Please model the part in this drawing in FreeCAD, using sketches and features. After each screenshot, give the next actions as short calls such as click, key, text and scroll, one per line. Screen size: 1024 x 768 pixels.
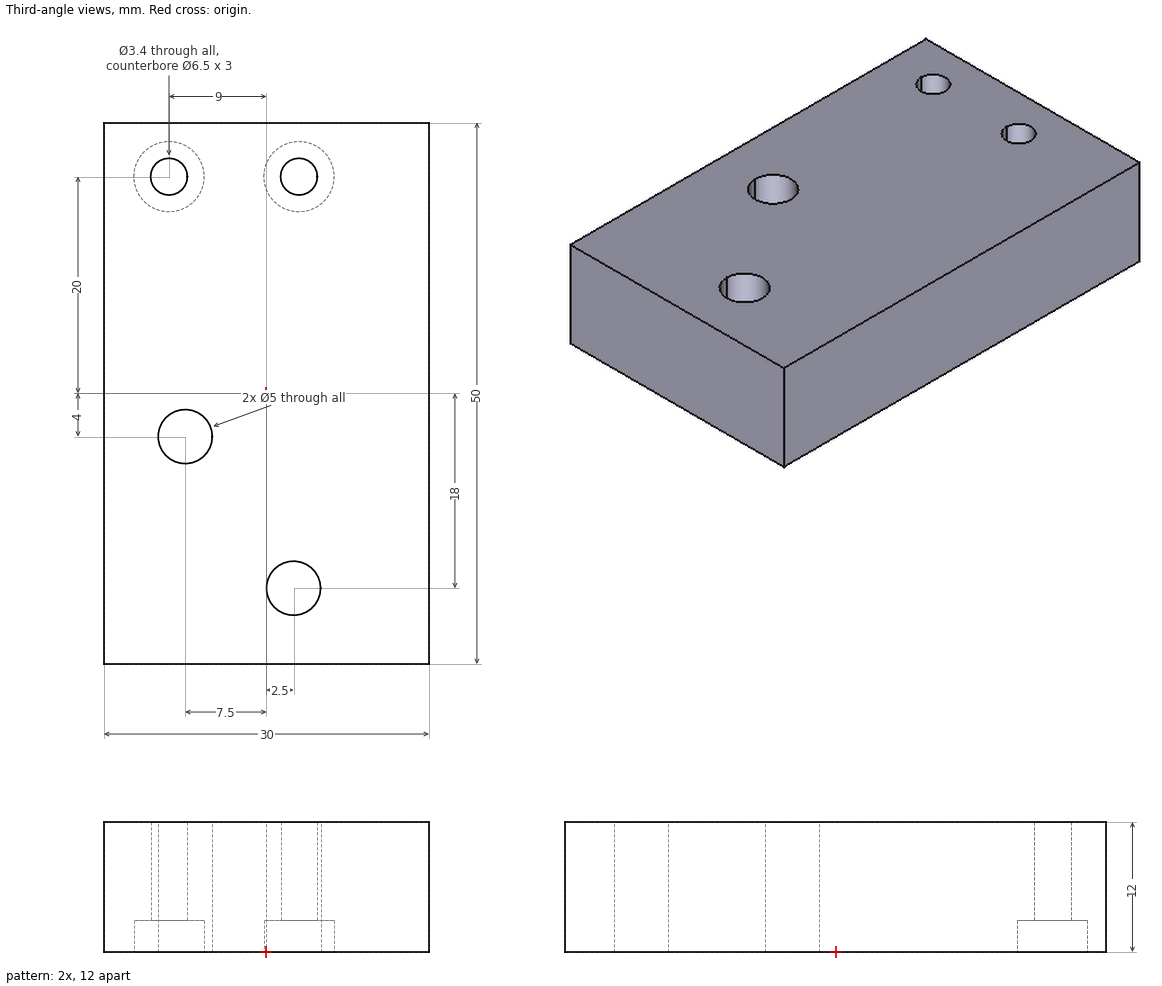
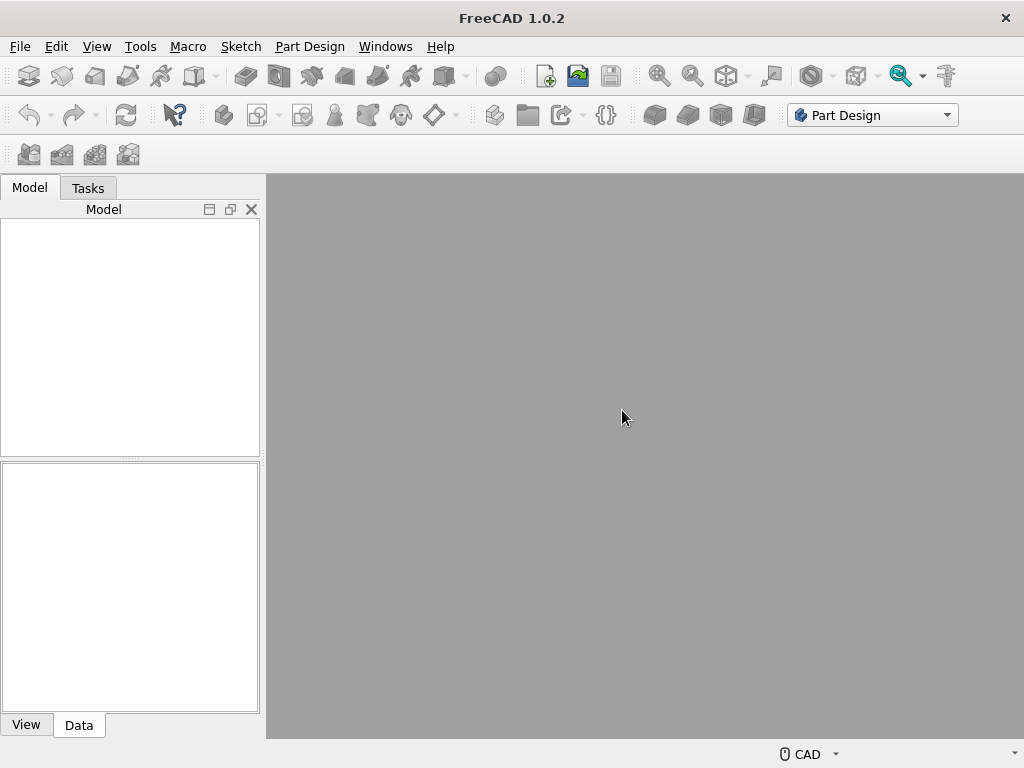
key(ctrl+n)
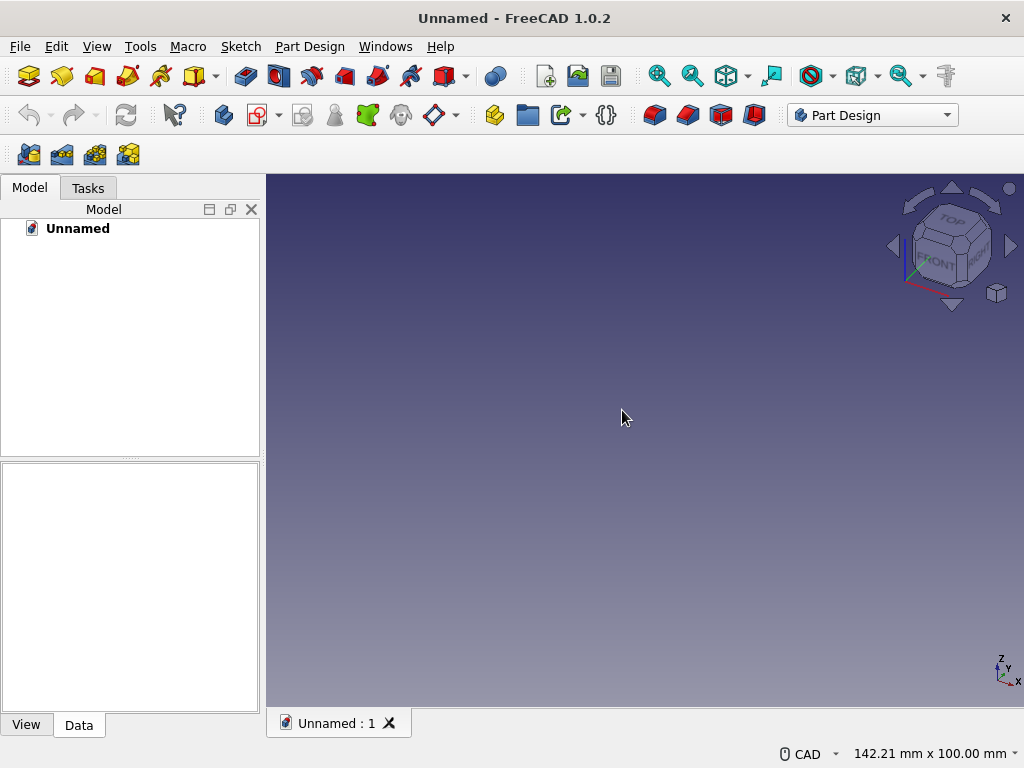
click(256, 116)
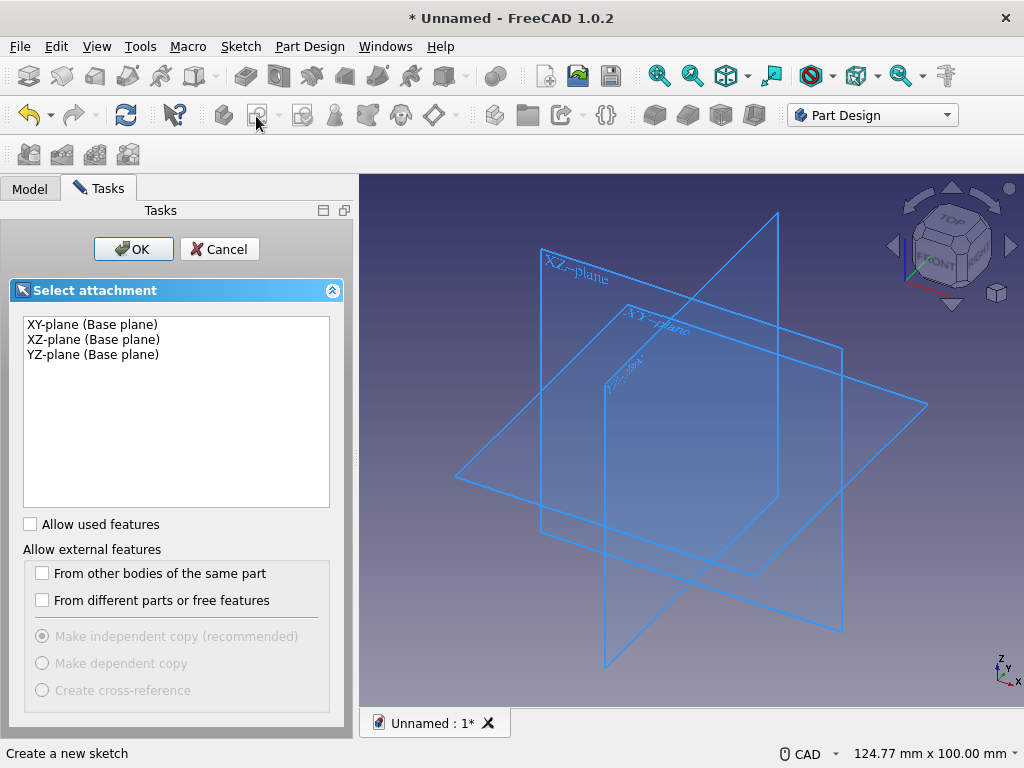
click(84, 324)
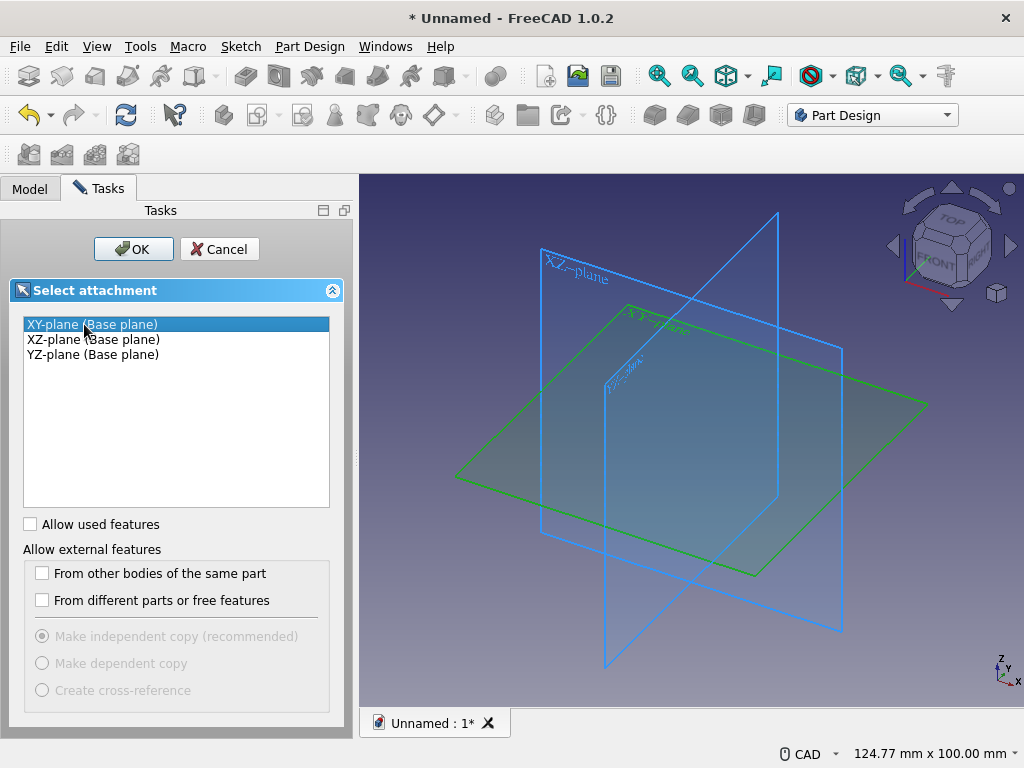
click(134, 249)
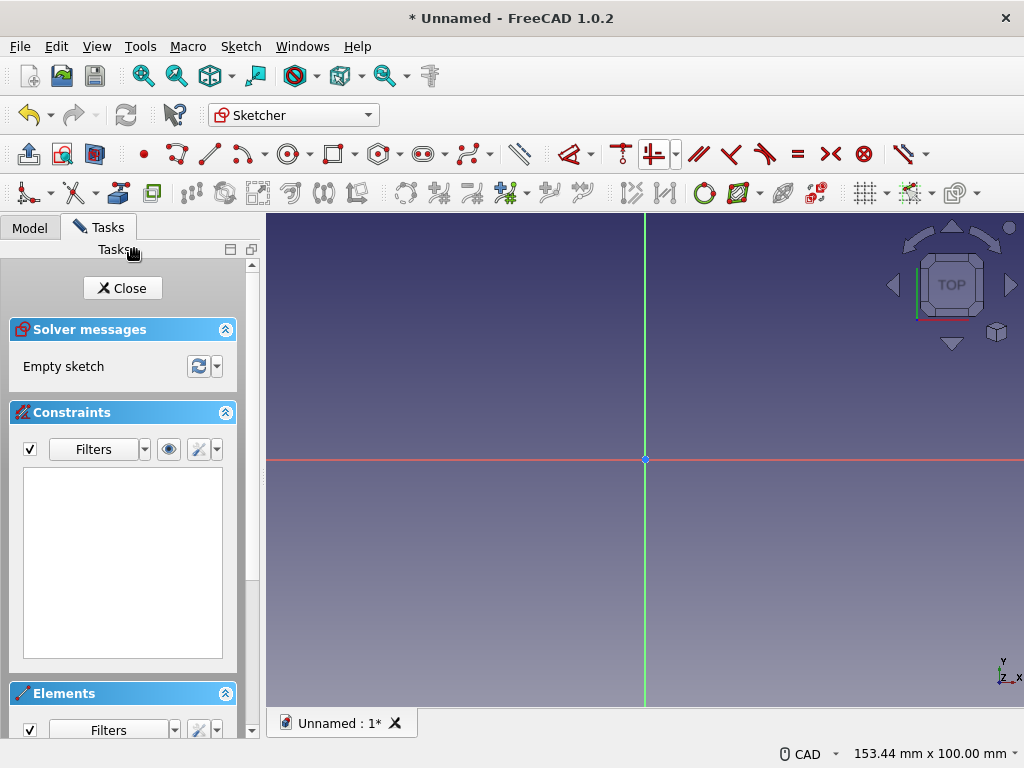
key(g)
key(v)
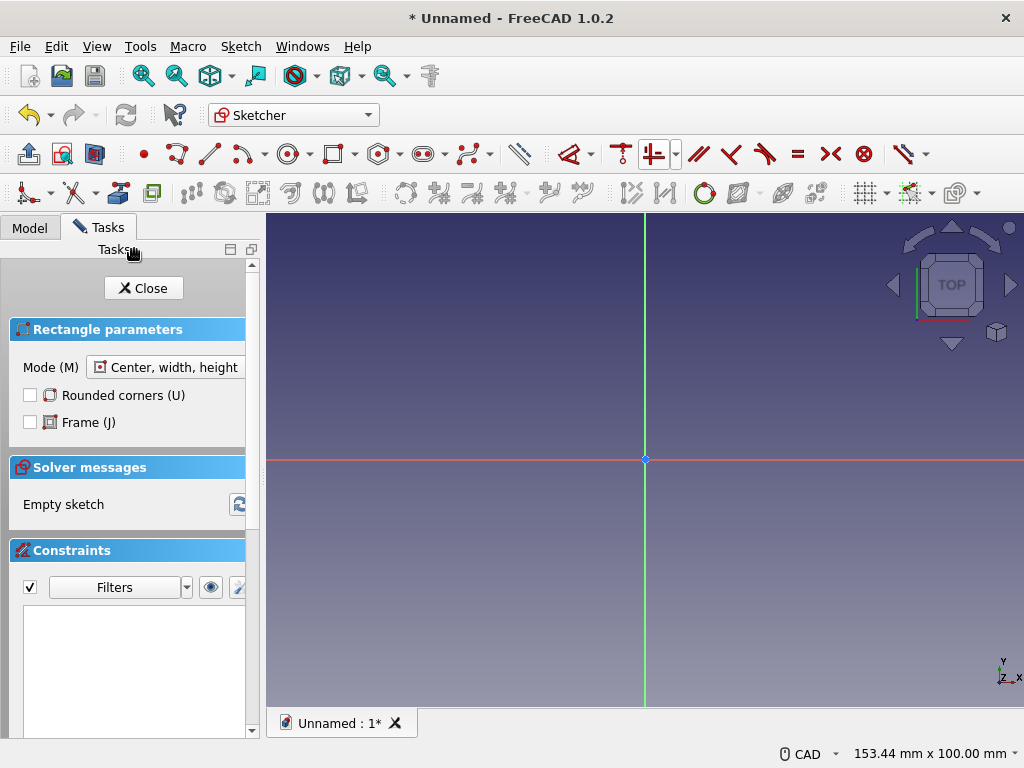
click(645, 460)
move(719, 336)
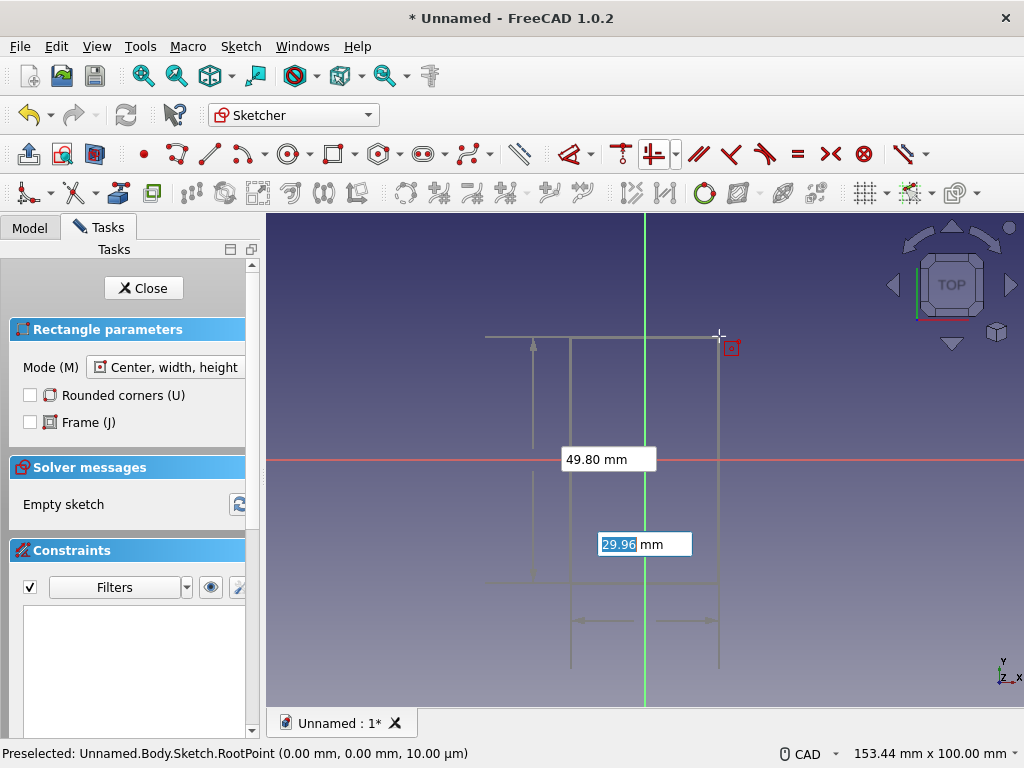
text(30)
key(Tab)
text(50)
key(Return)
key(Escape)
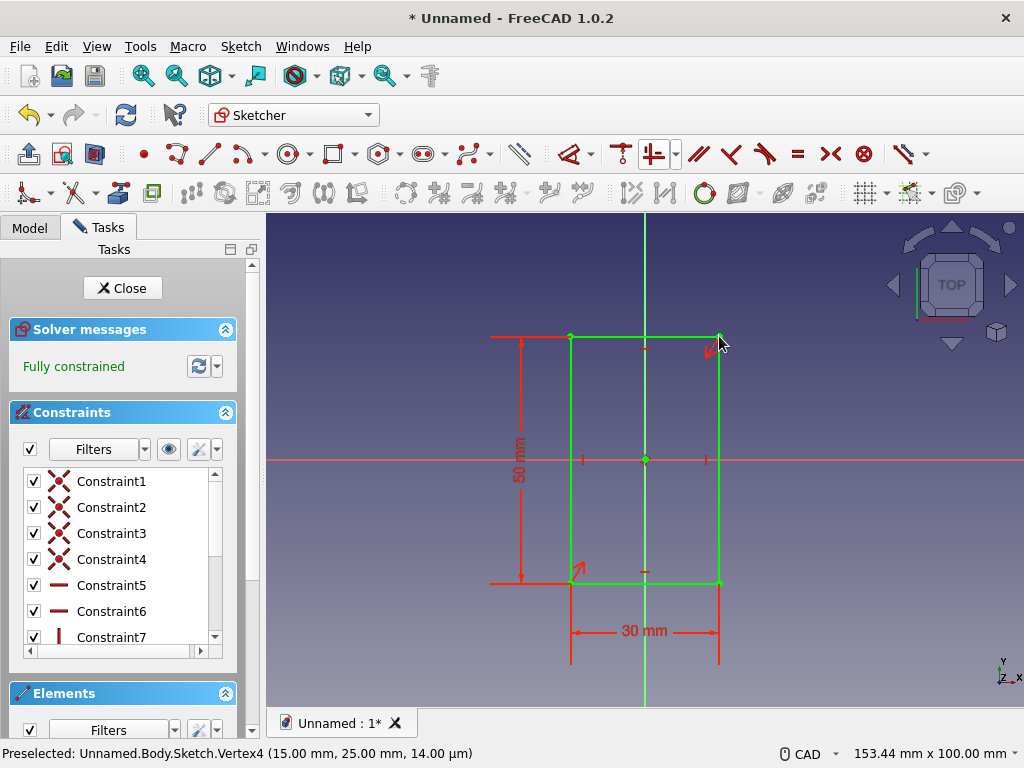
click(123, 288)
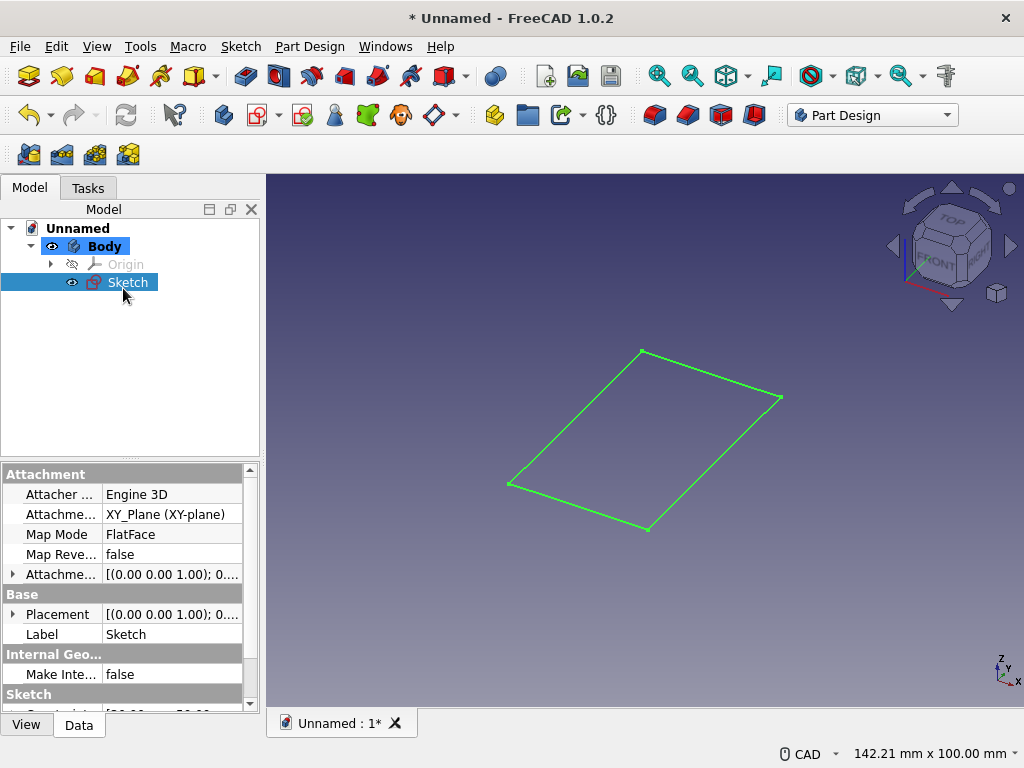
click(29, 76)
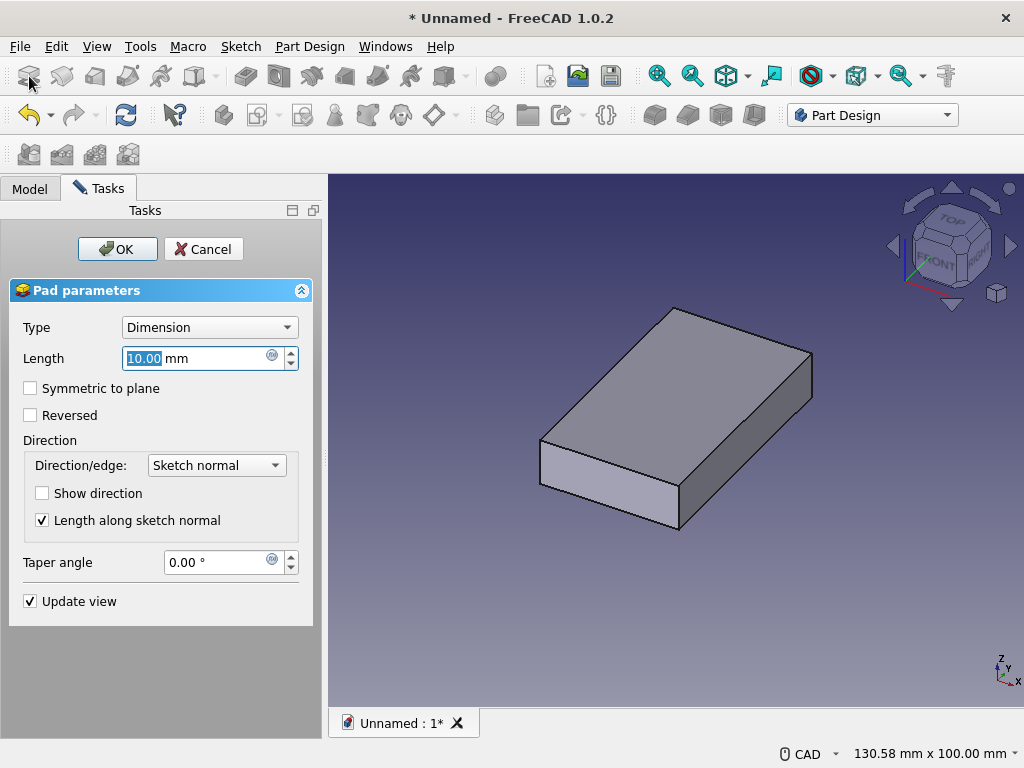
text(12)
key(Tab)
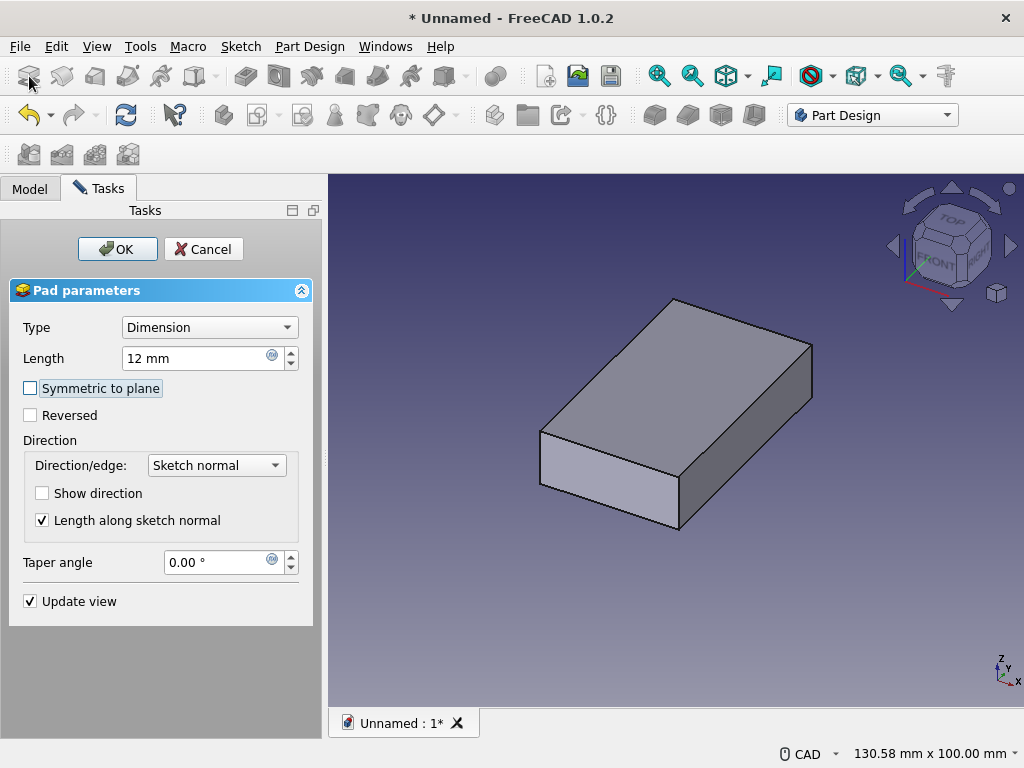
click(118, 249)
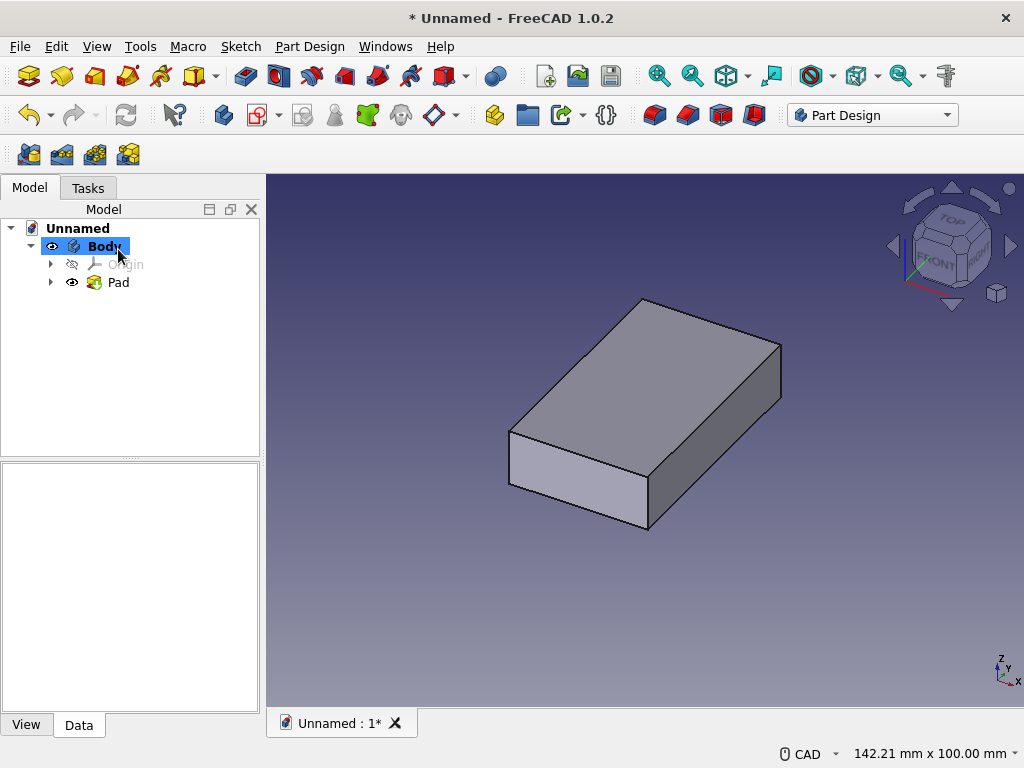
click(660, 76)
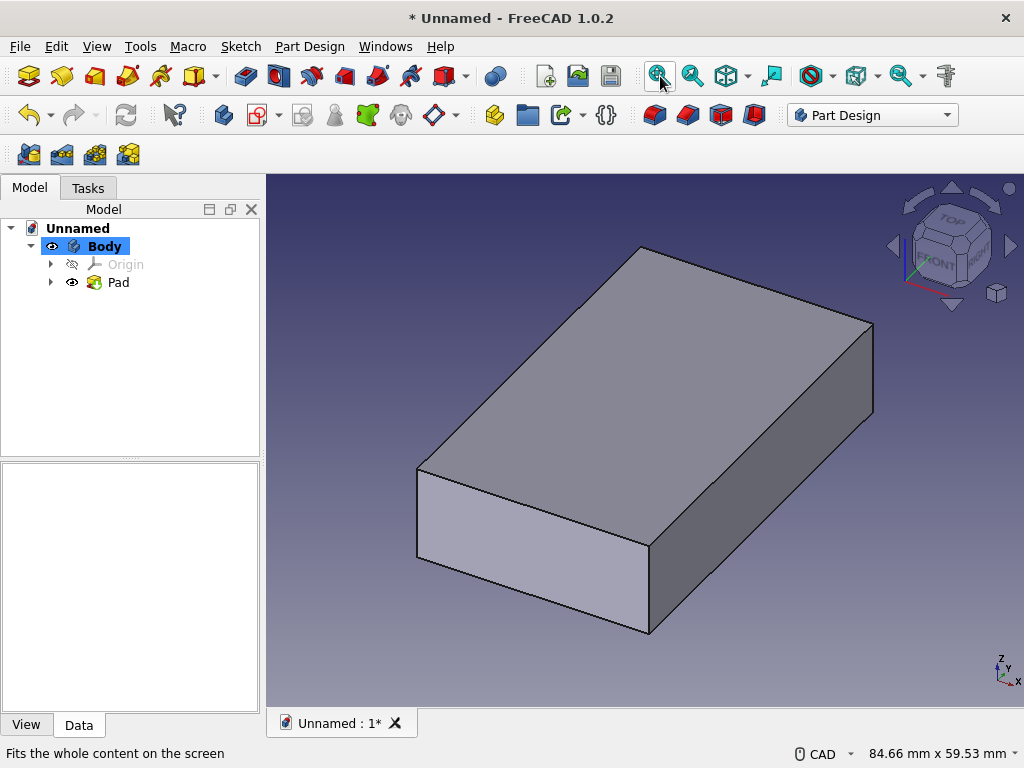
key(5)